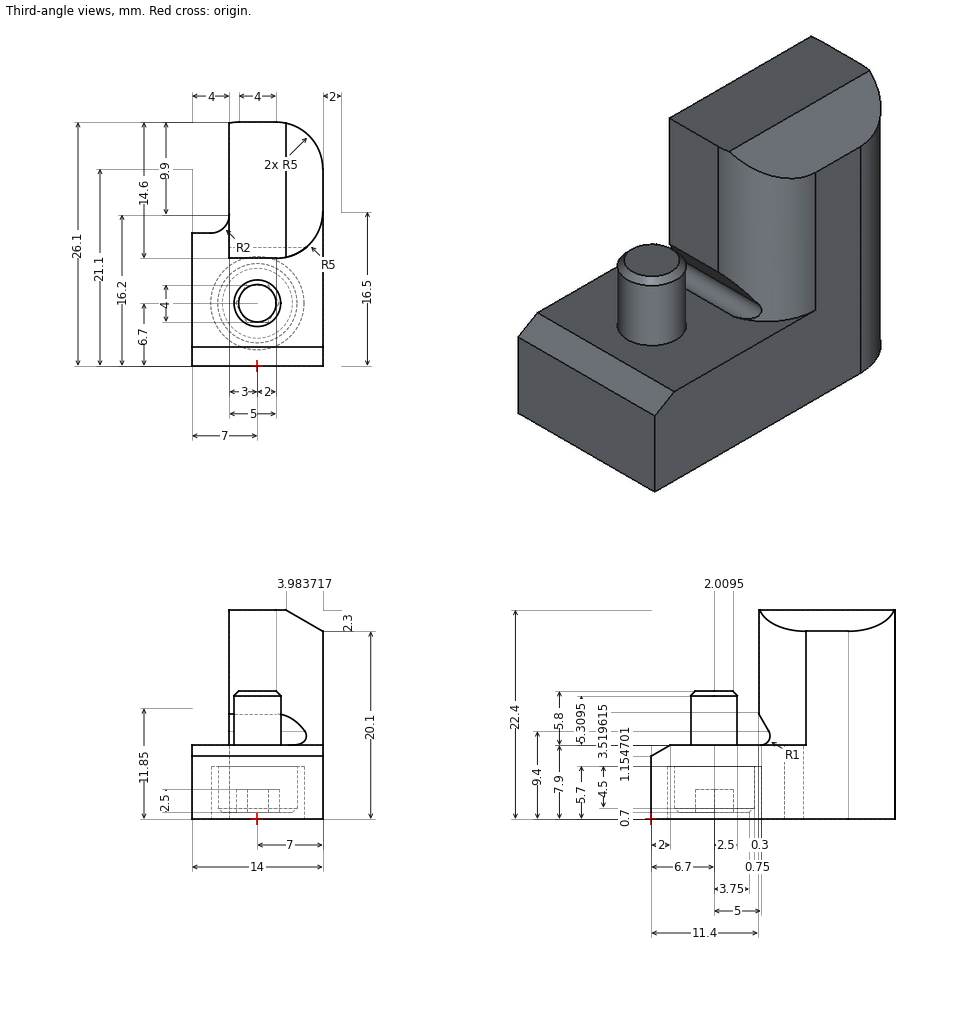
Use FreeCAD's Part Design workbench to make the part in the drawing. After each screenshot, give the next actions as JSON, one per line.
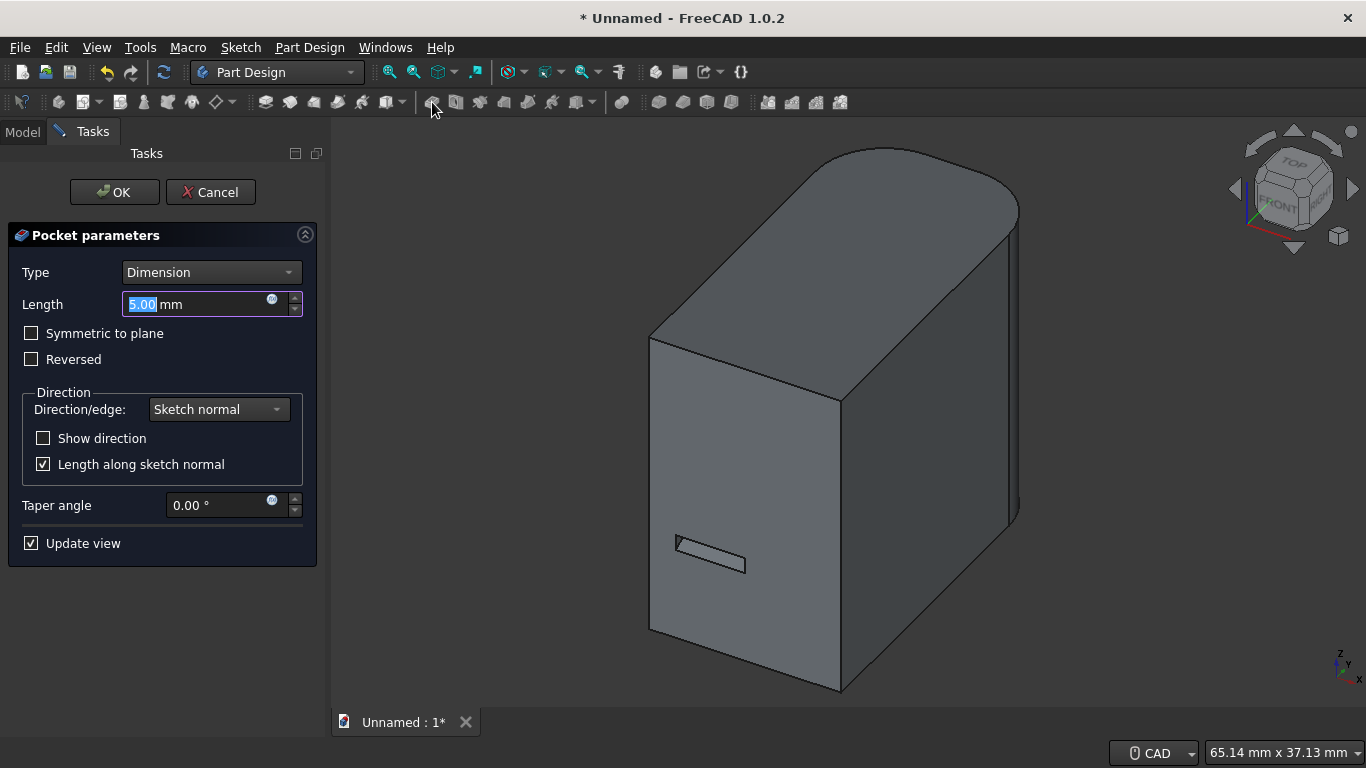
{"action": "type", "text": "14"}
{"action": "key", "text": "Tab"}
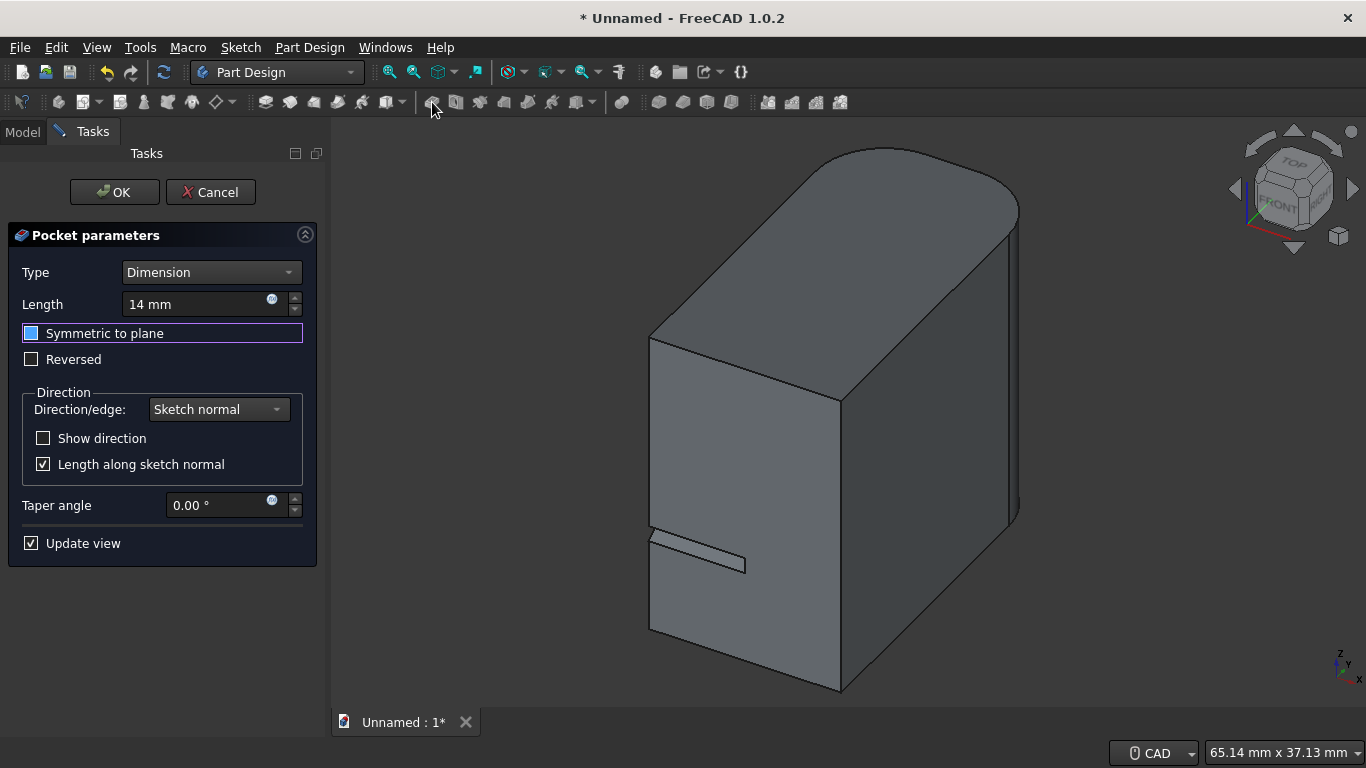
{"action": "left_click", "coordinate": [30, 333]}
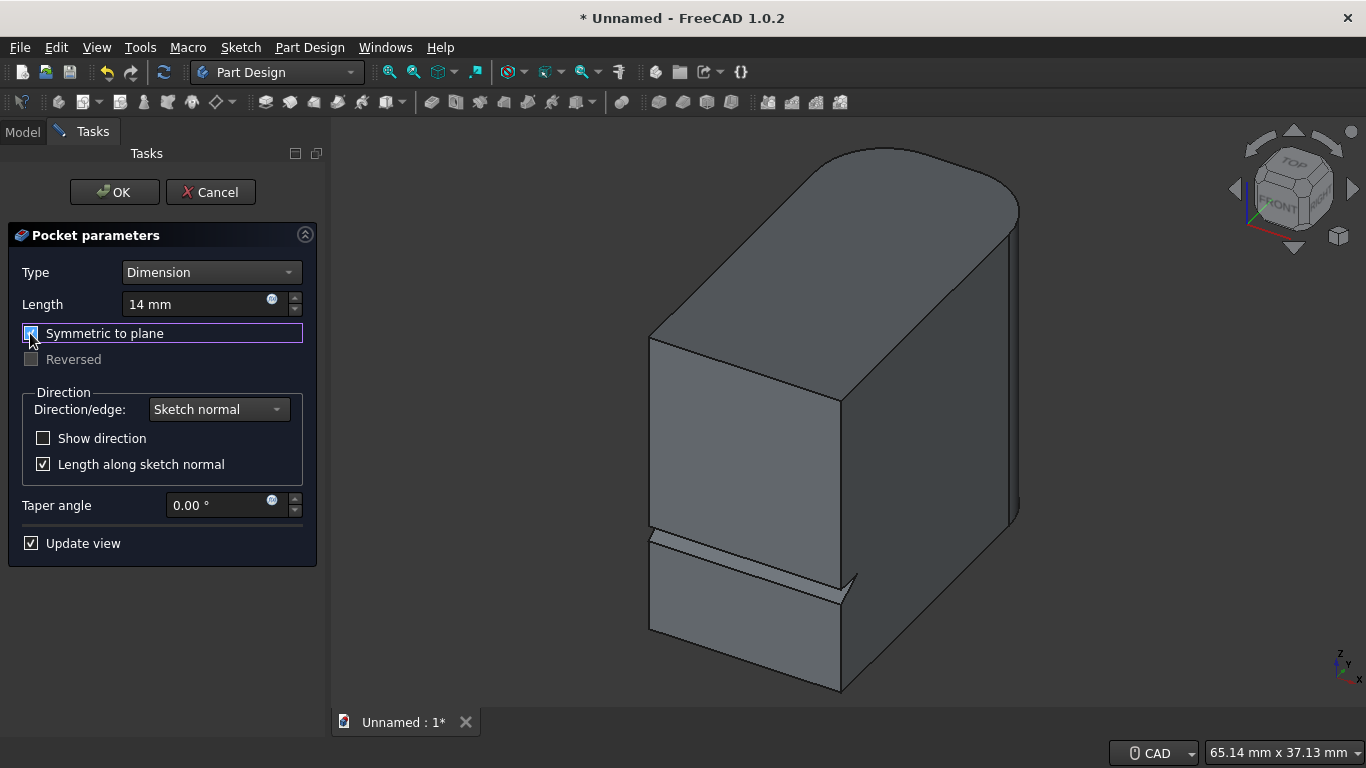
{"action": "left_click", "coordinate": [115, 192]}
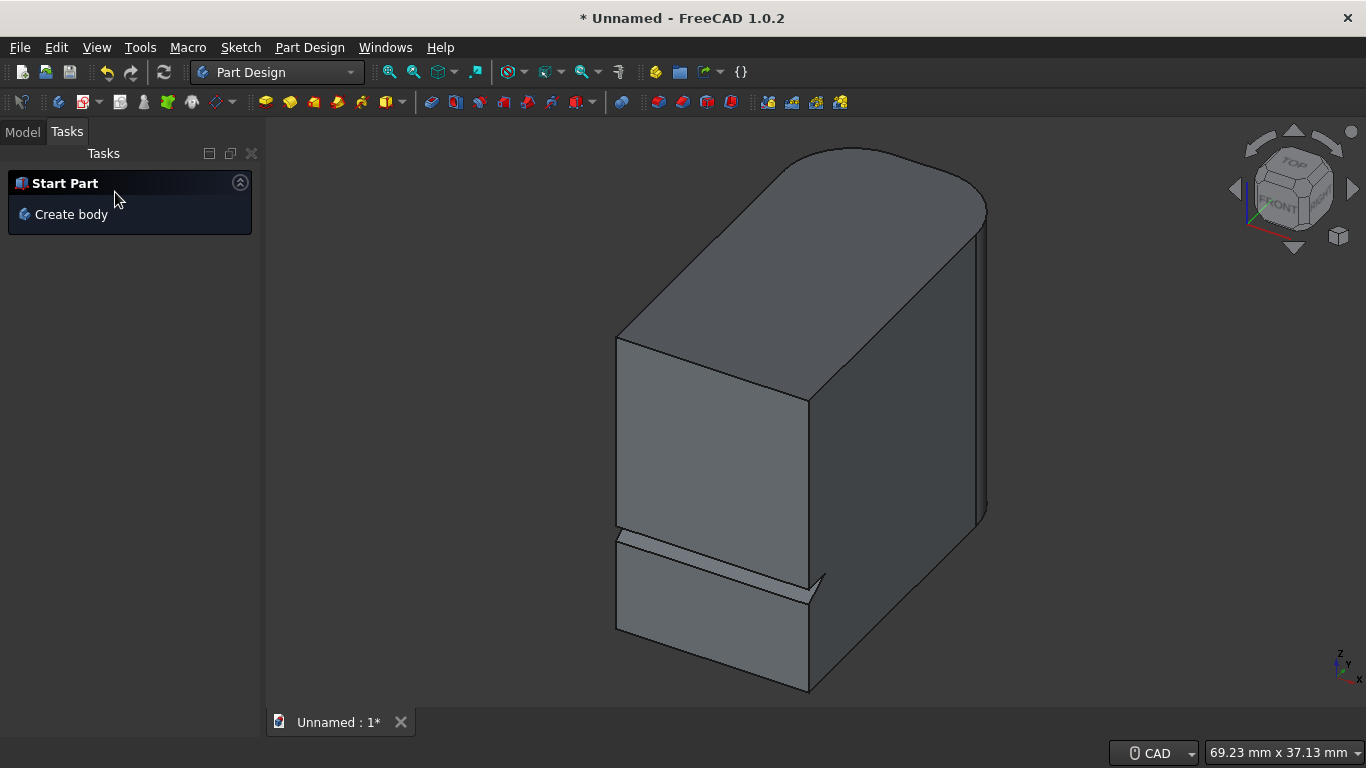
{"action": "left_click", "coordinate": [23, 131]}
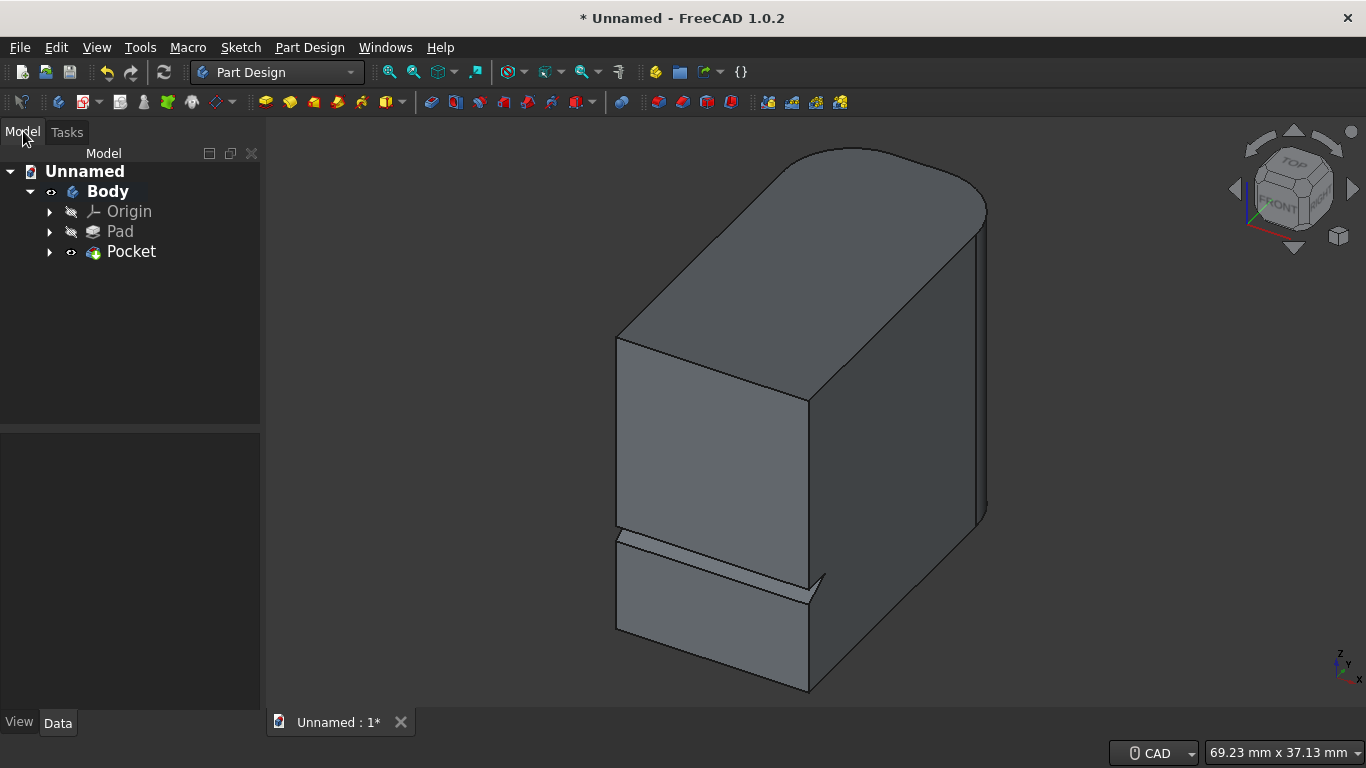
{"action": "left_click", "coordinate": [50, 212]}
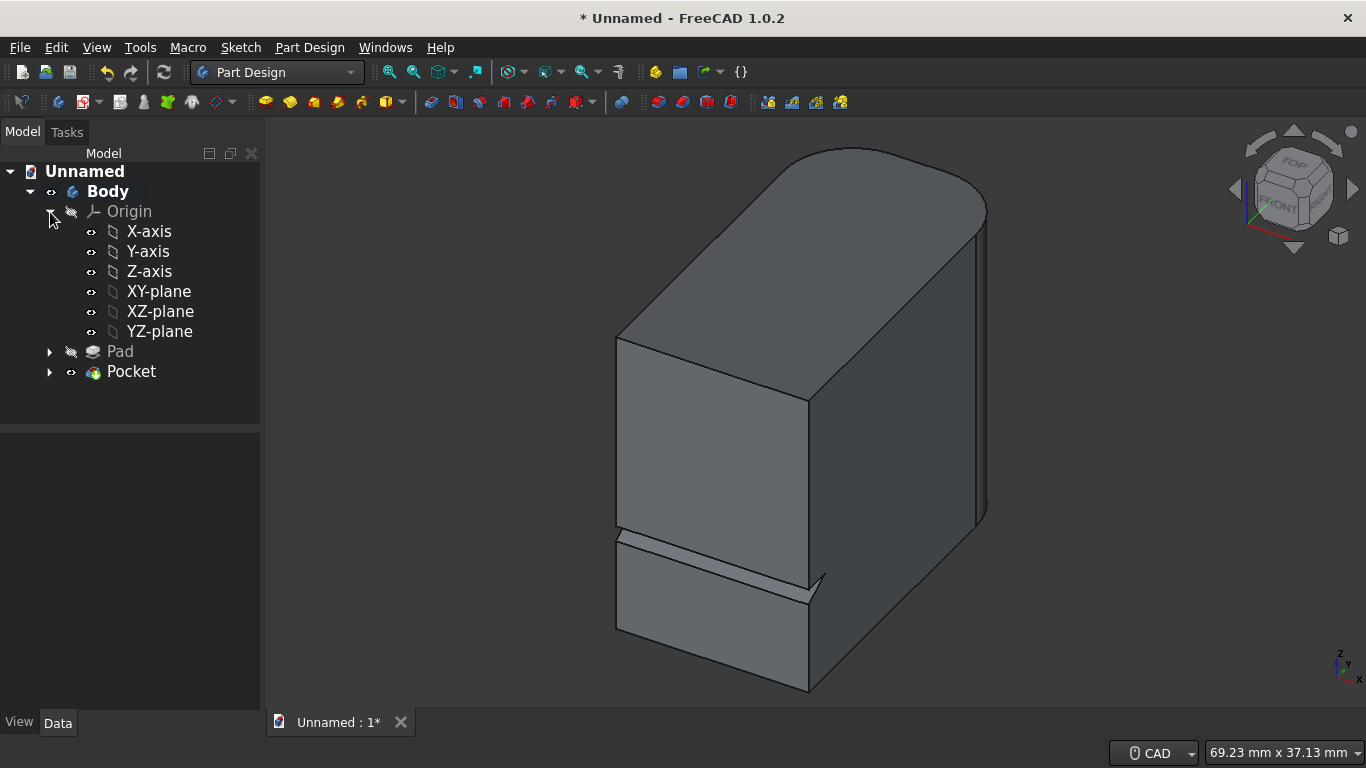
{"action": "left_click", "coordinate": [136, 292]}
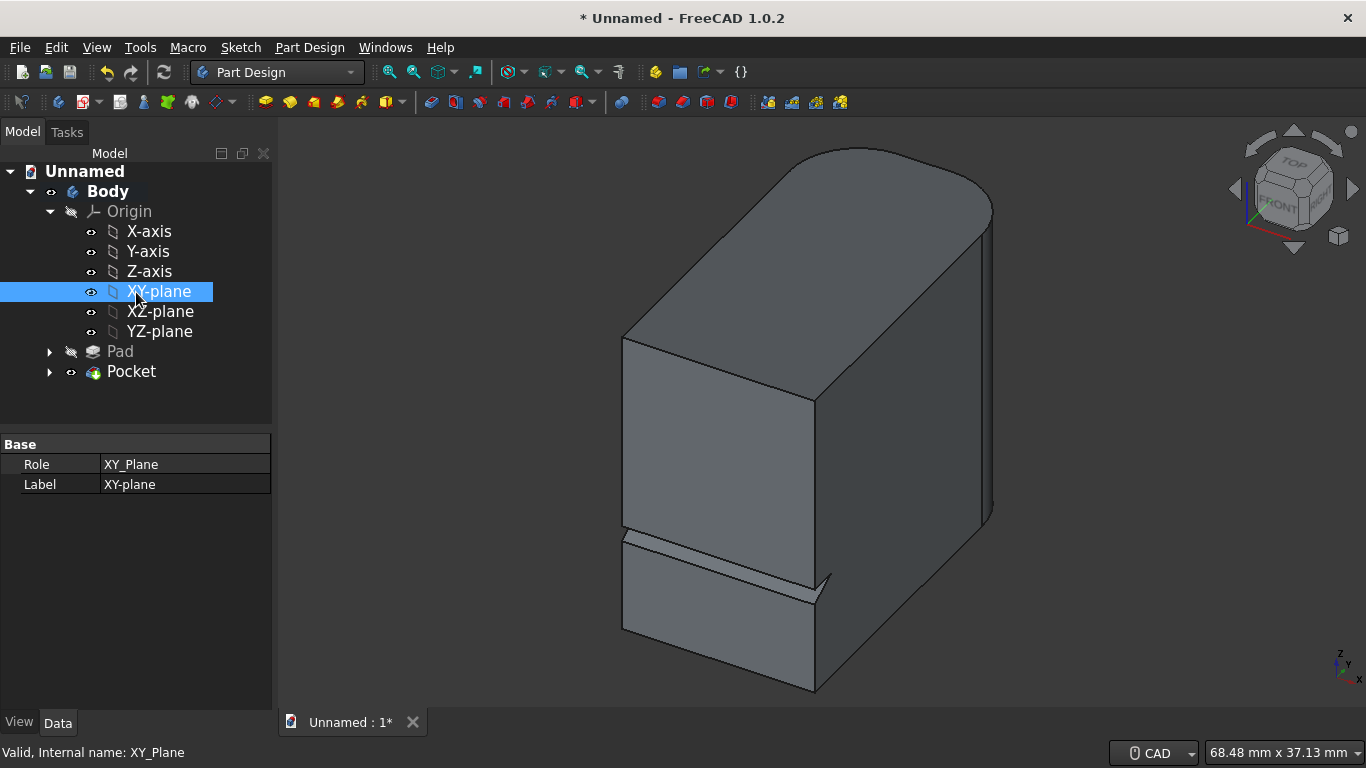
{"action": "left_click", "coordinate": [216, 102]}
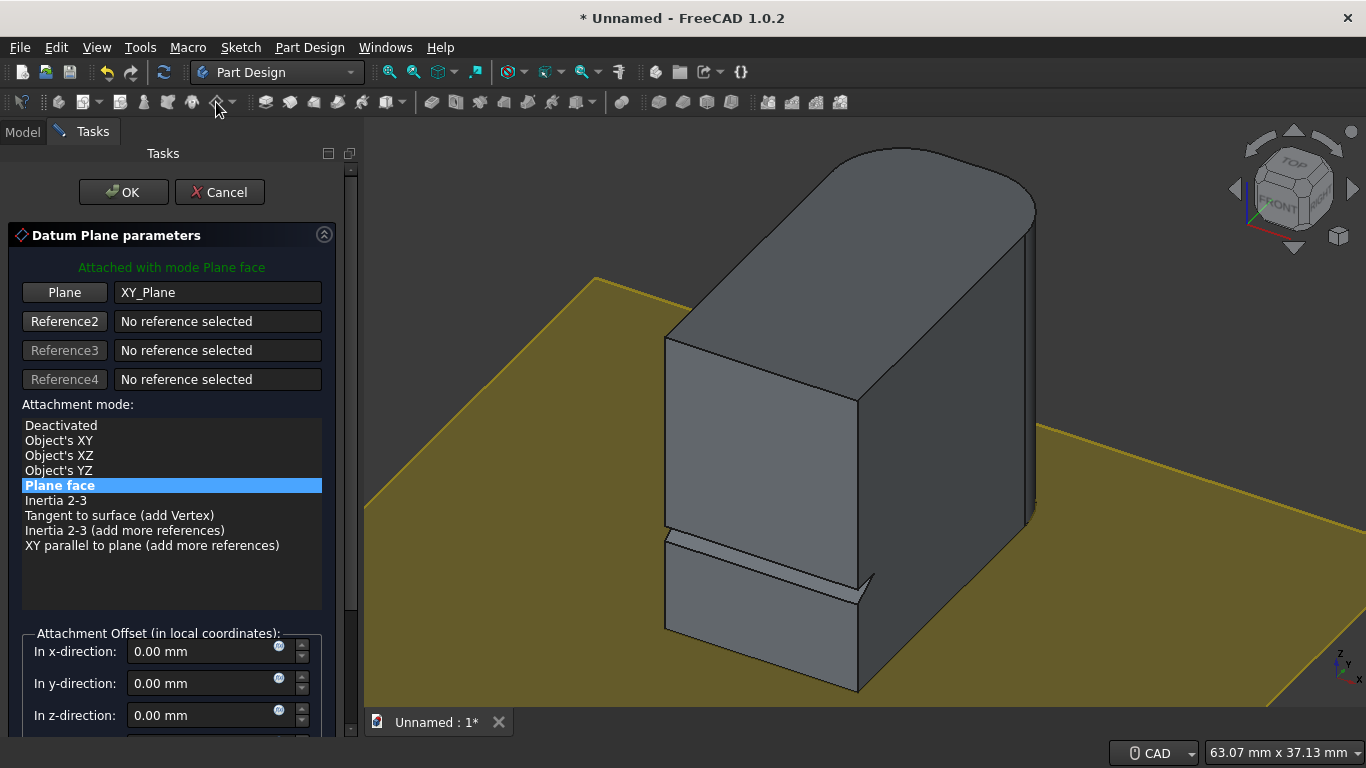
{"action": "triple_click", "coordinate": [210, 715]}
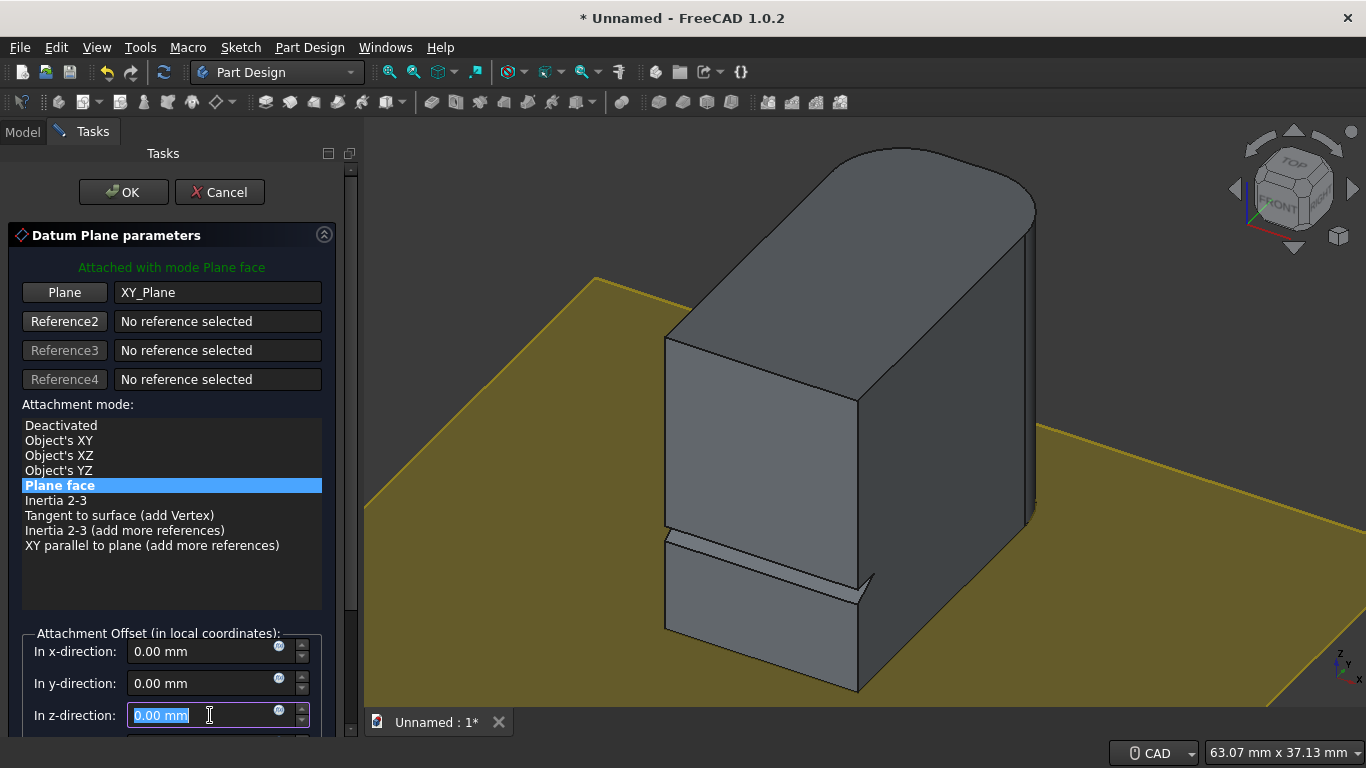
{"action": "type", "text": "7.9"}
{"action": "key", "text": "Tab"}